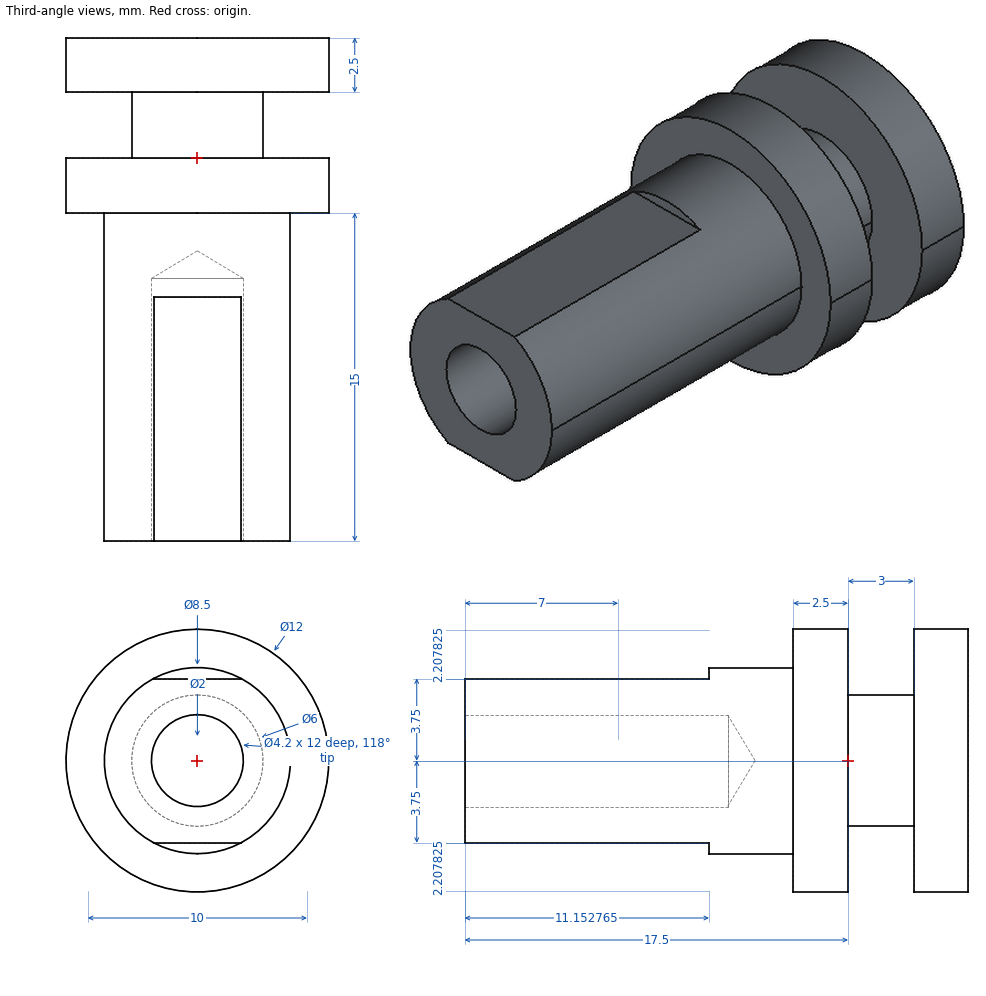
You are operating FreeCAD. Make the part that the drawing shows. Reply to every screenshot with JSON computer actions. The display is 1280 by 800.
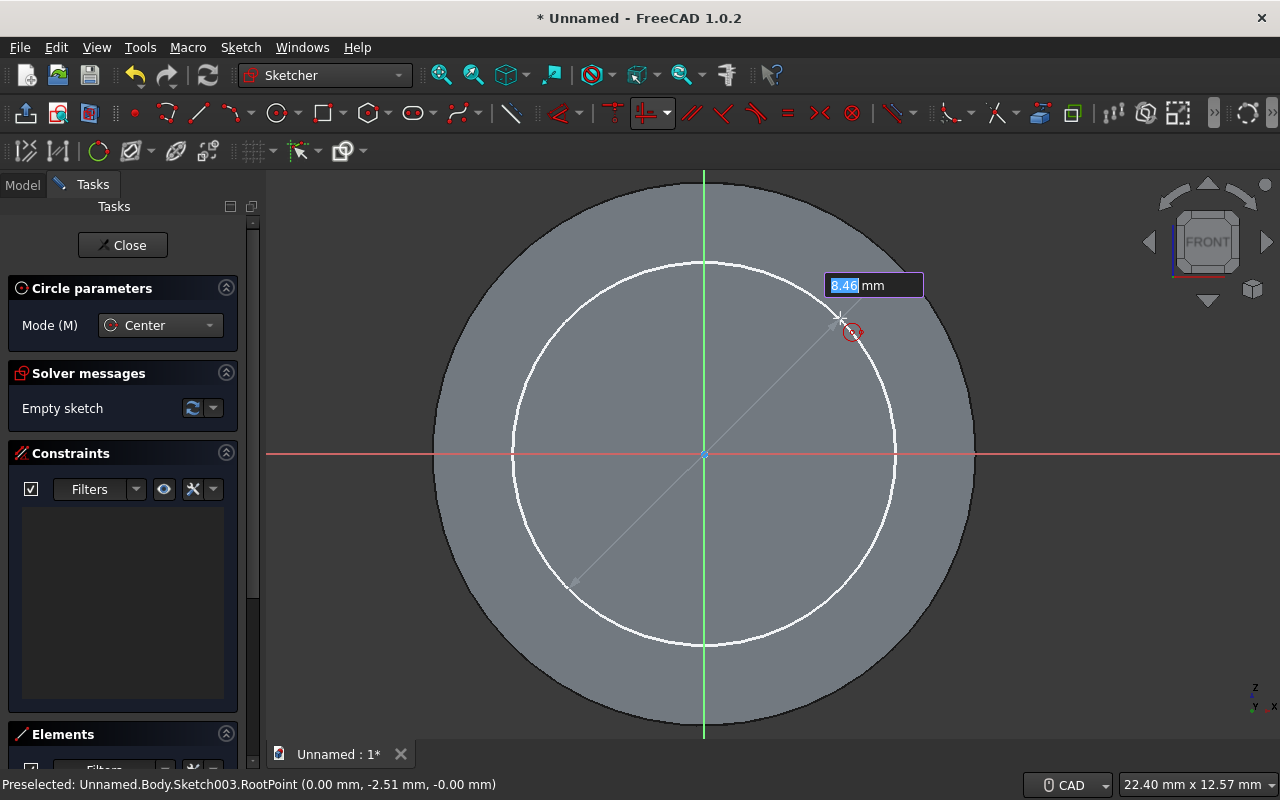
{"action": "type", "text": "8.5"}
{"action": "key", "text": "Return"}
{"action": "key", "text": "Escape"}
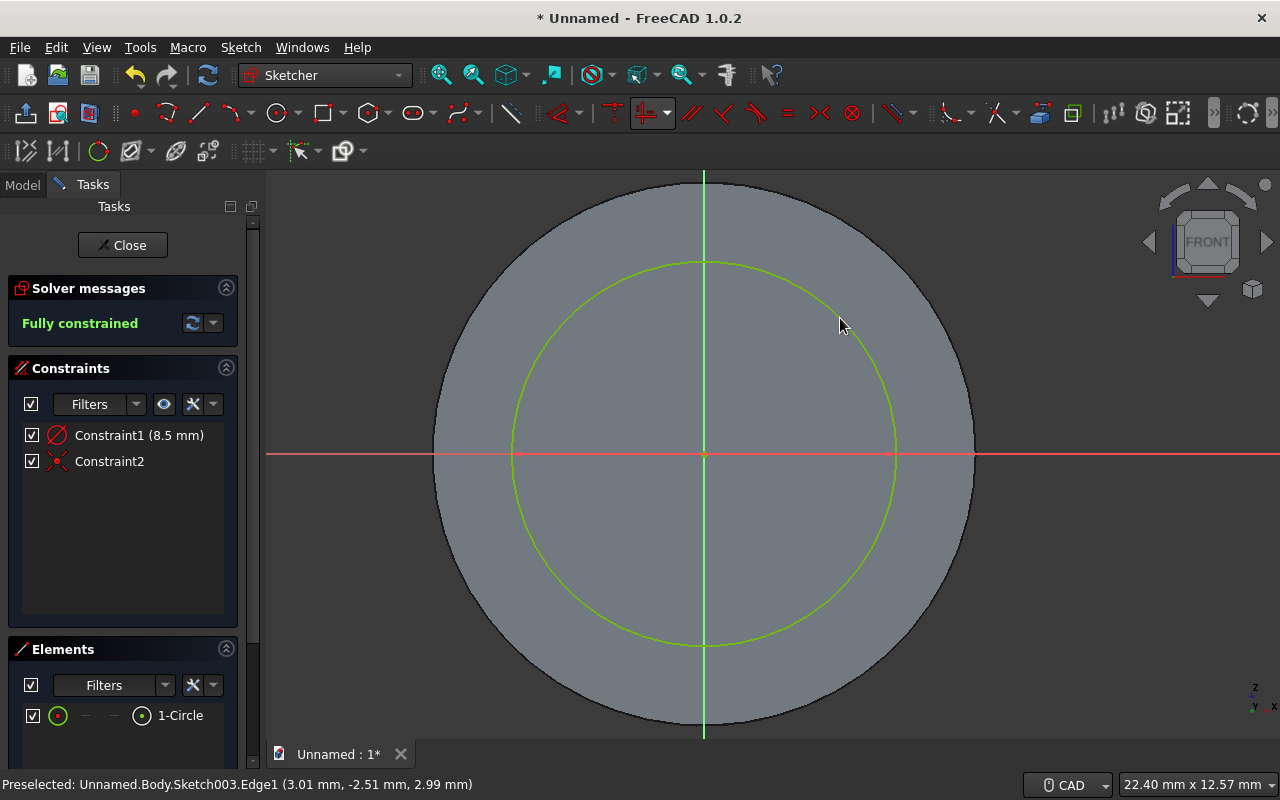
{"action": "left_click", "coordinate": [123, 245]}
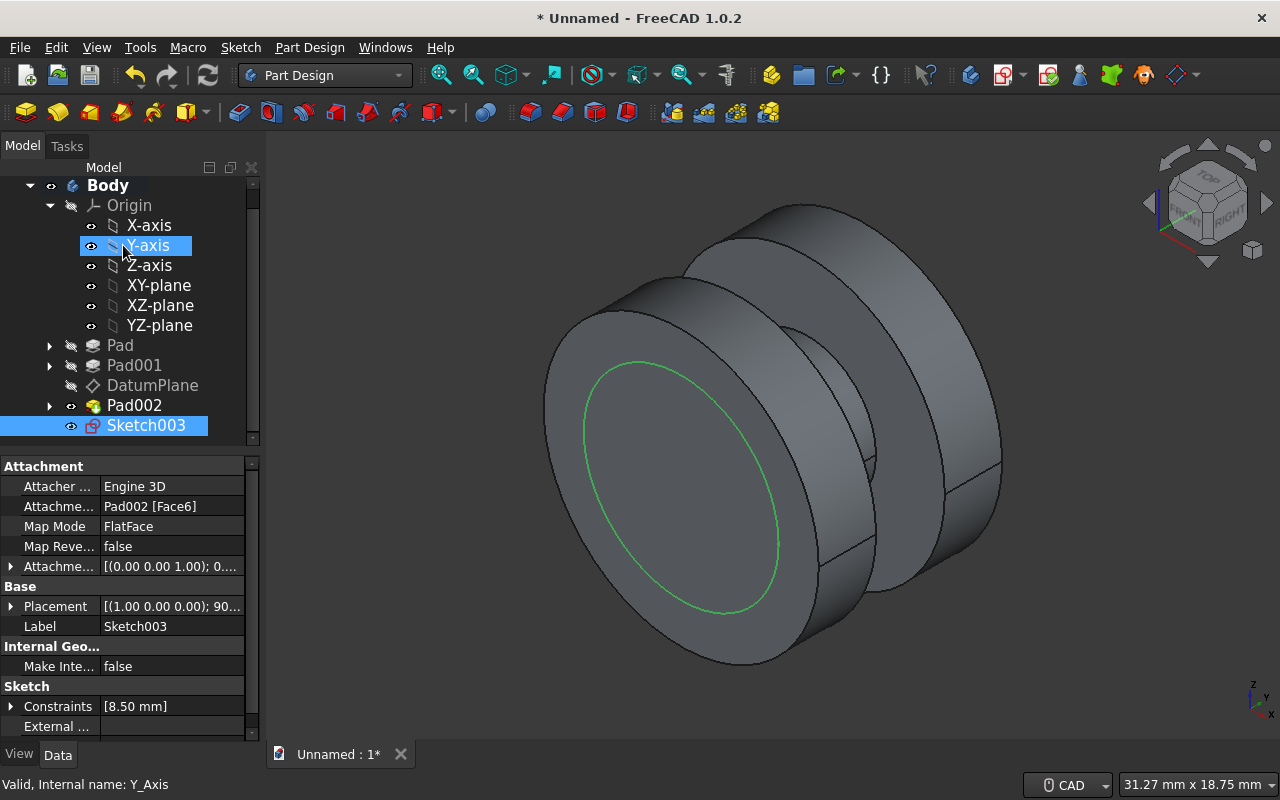
{"action": "left_click", "coordinate": [26, 112]}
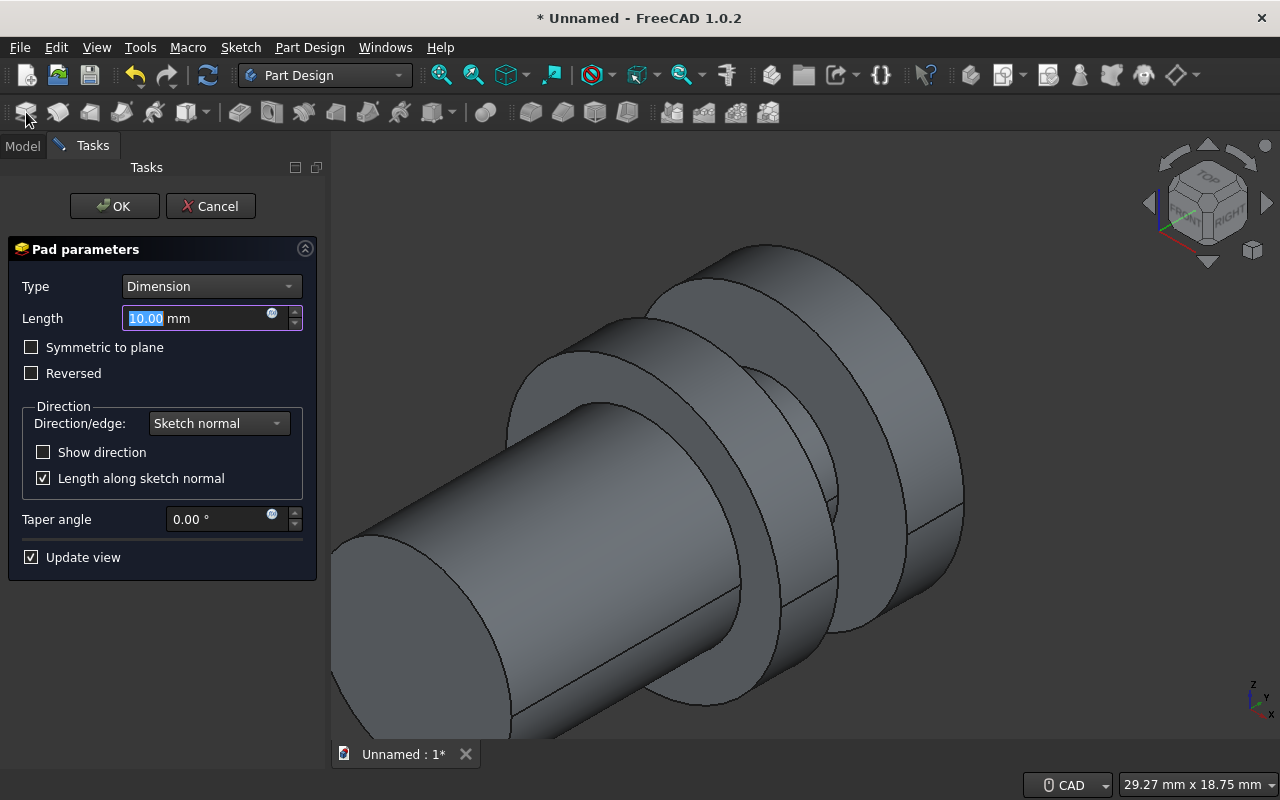
{"action": "type", "text": "15"}
{"action": "key", "text": "Tab"}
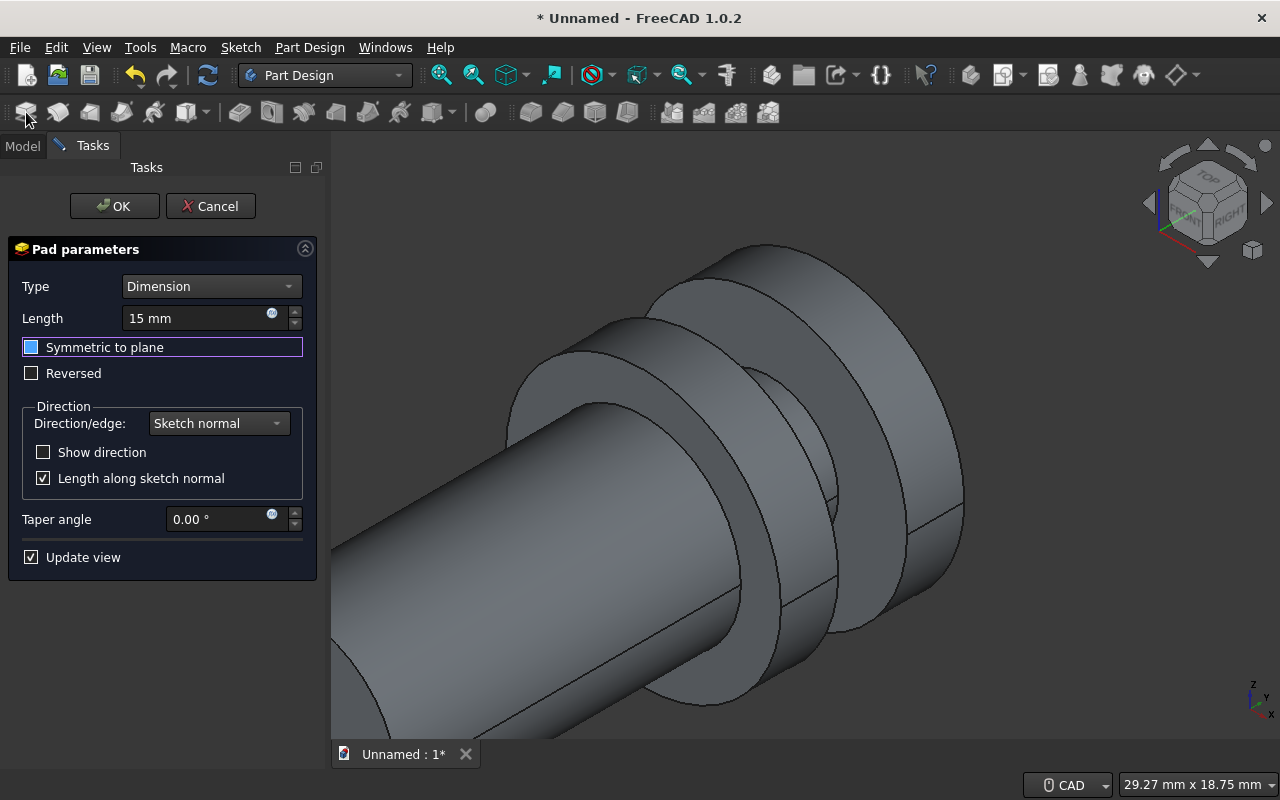
{"action": "left_click", "coordinate": [115, 206]}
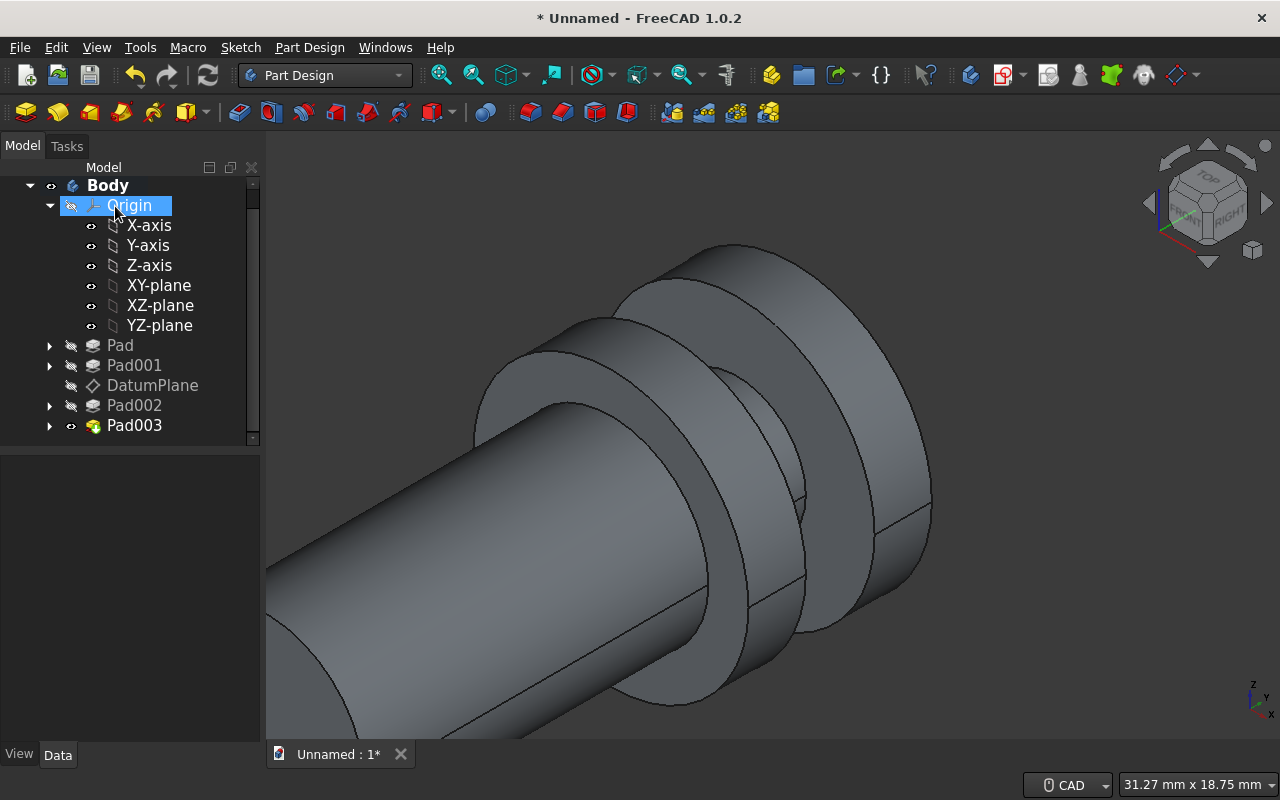
{"action": "key", "text": "v f"}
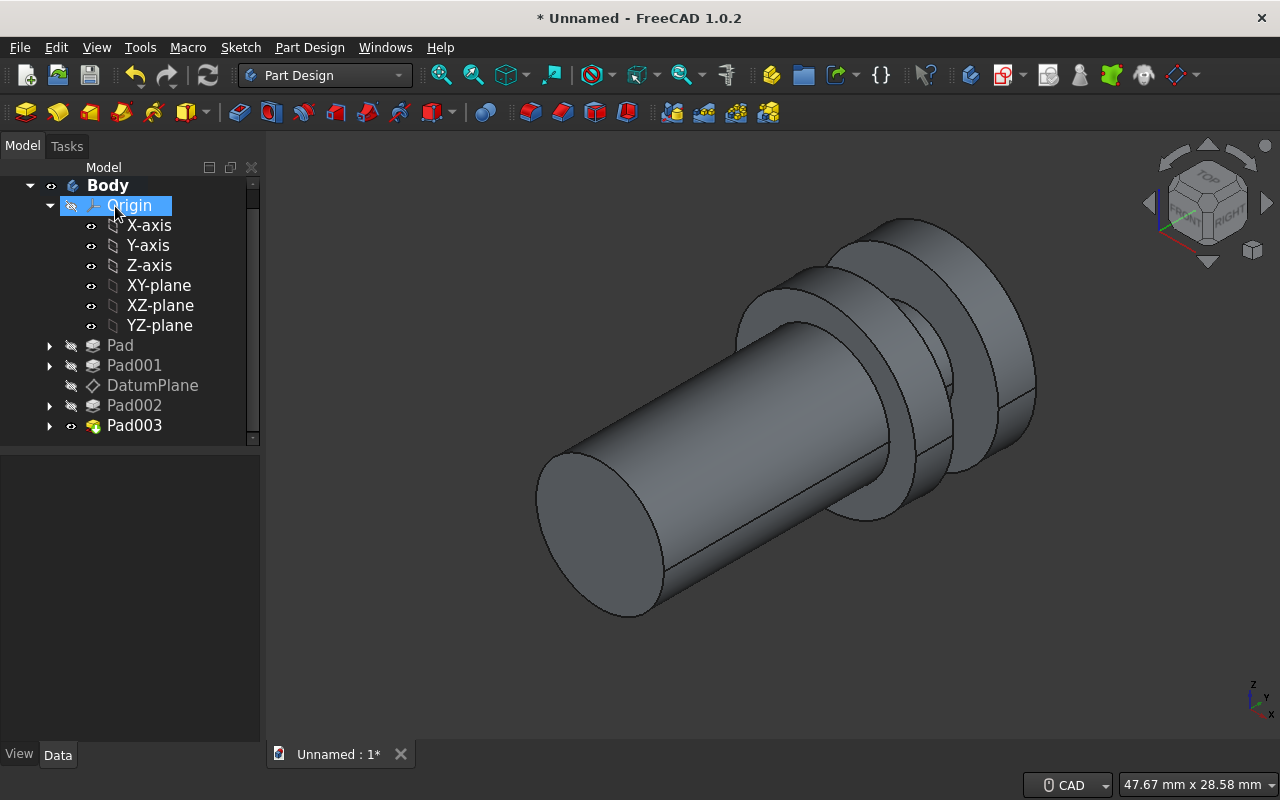
{"action": "left_click", "coordinate": [600, 534]}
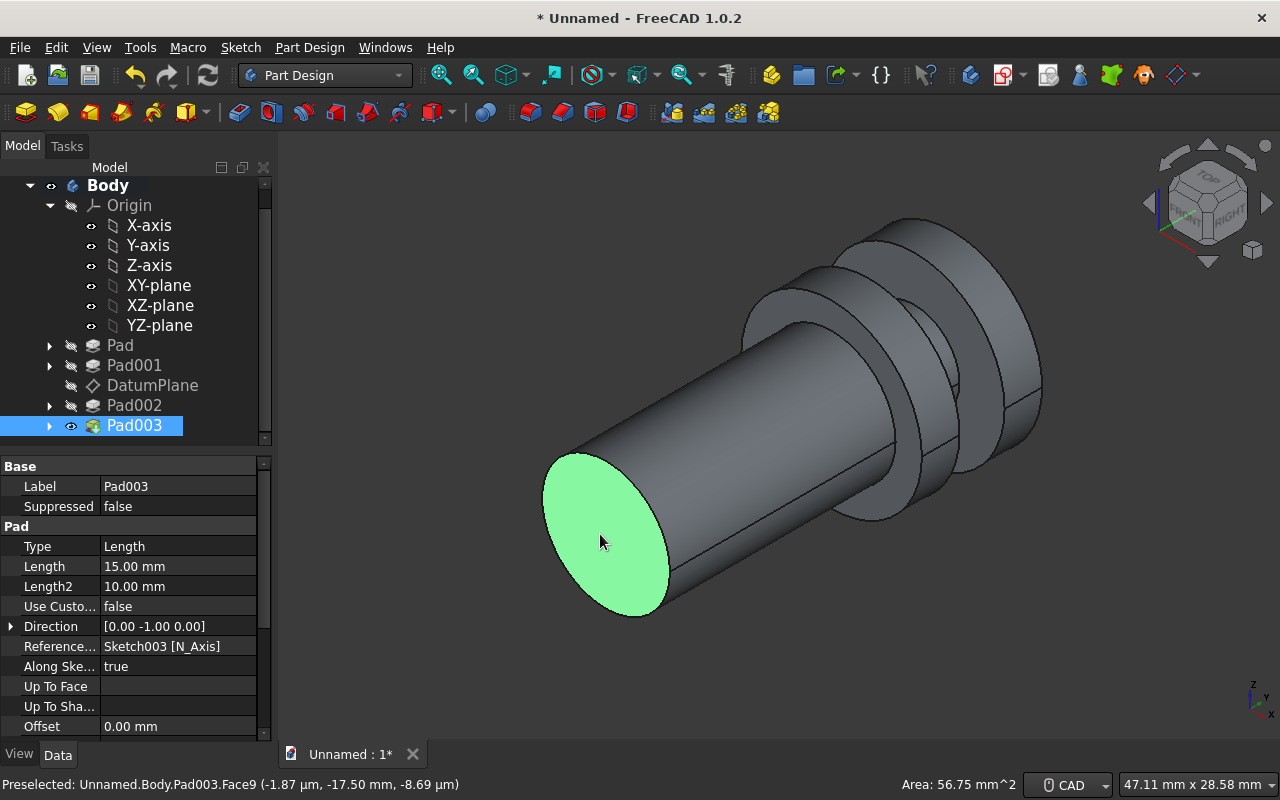
{"action": "left_click", "coordinate": [1004, 76]}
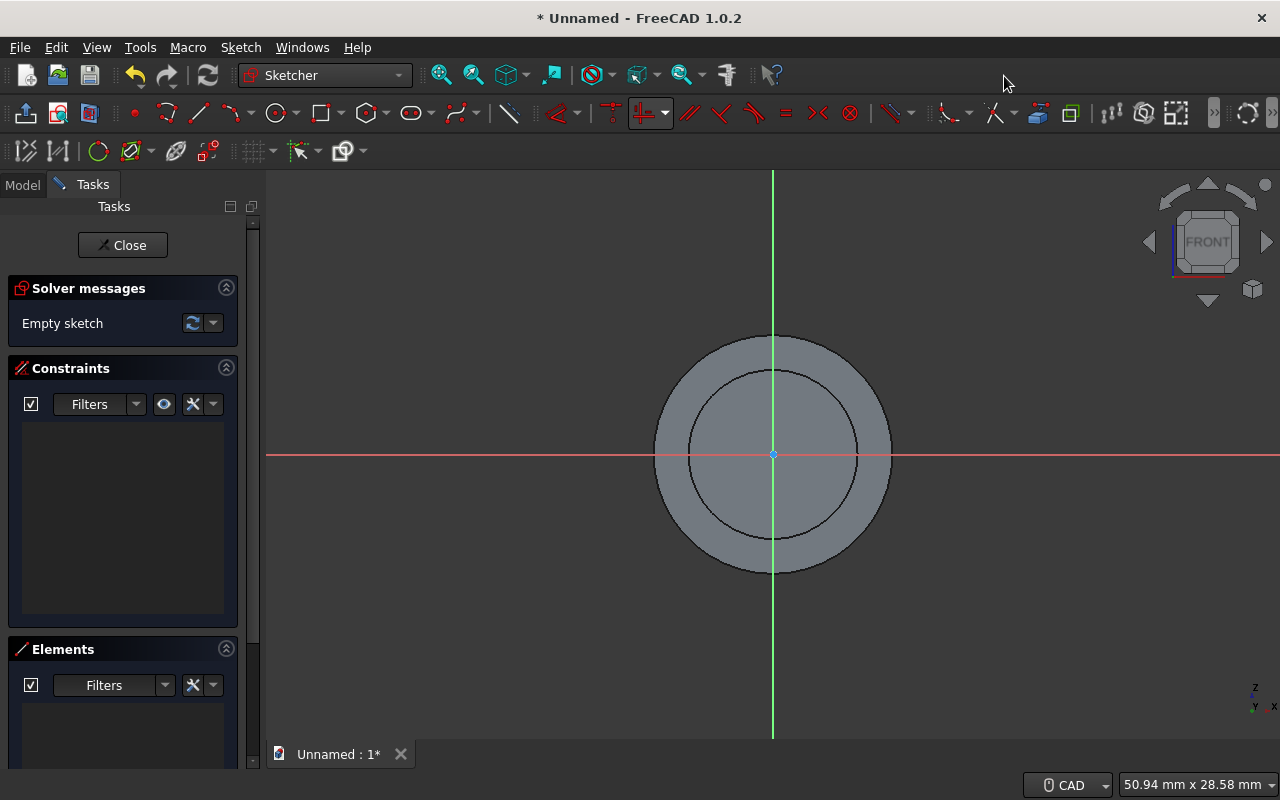
{"action": "scroll", "coordinate": [782, 454], "scroll_direction": "up", "scroll_amount": 11}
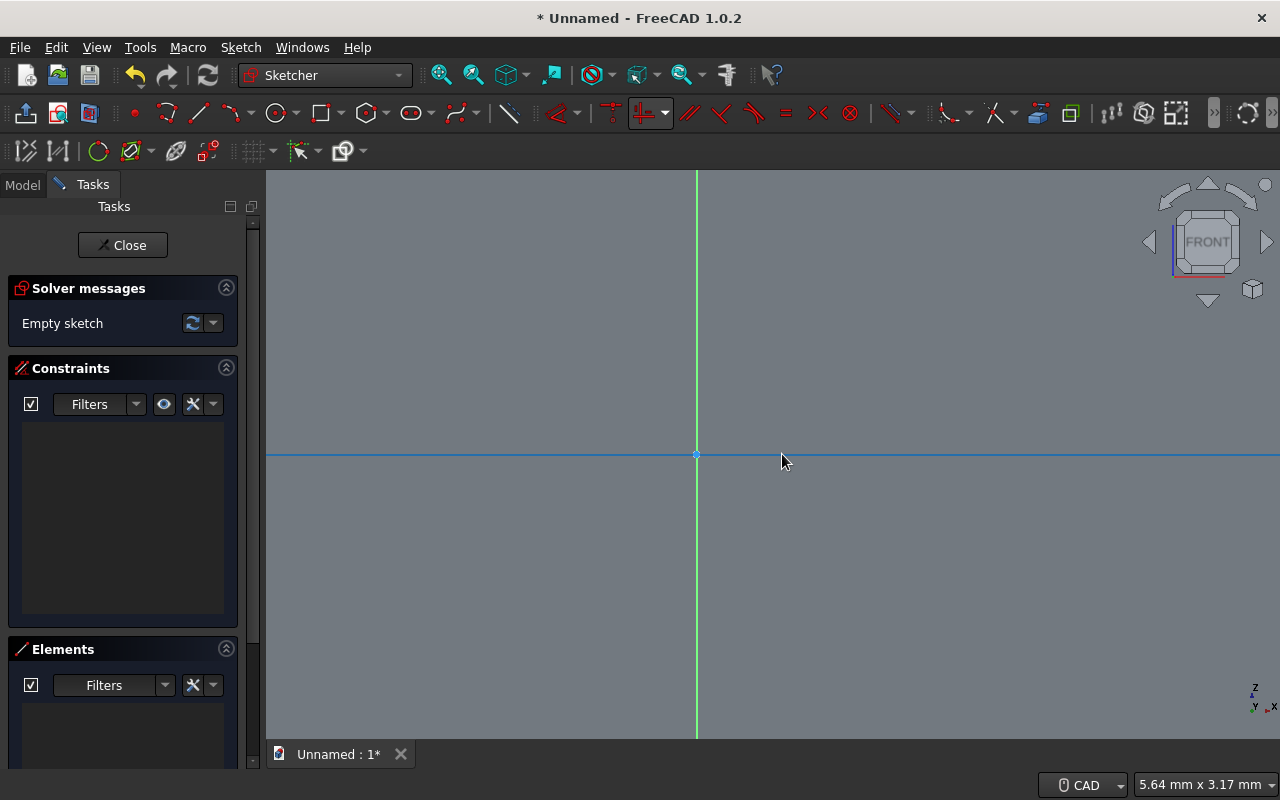
{"action": "key", "text": "g c"}